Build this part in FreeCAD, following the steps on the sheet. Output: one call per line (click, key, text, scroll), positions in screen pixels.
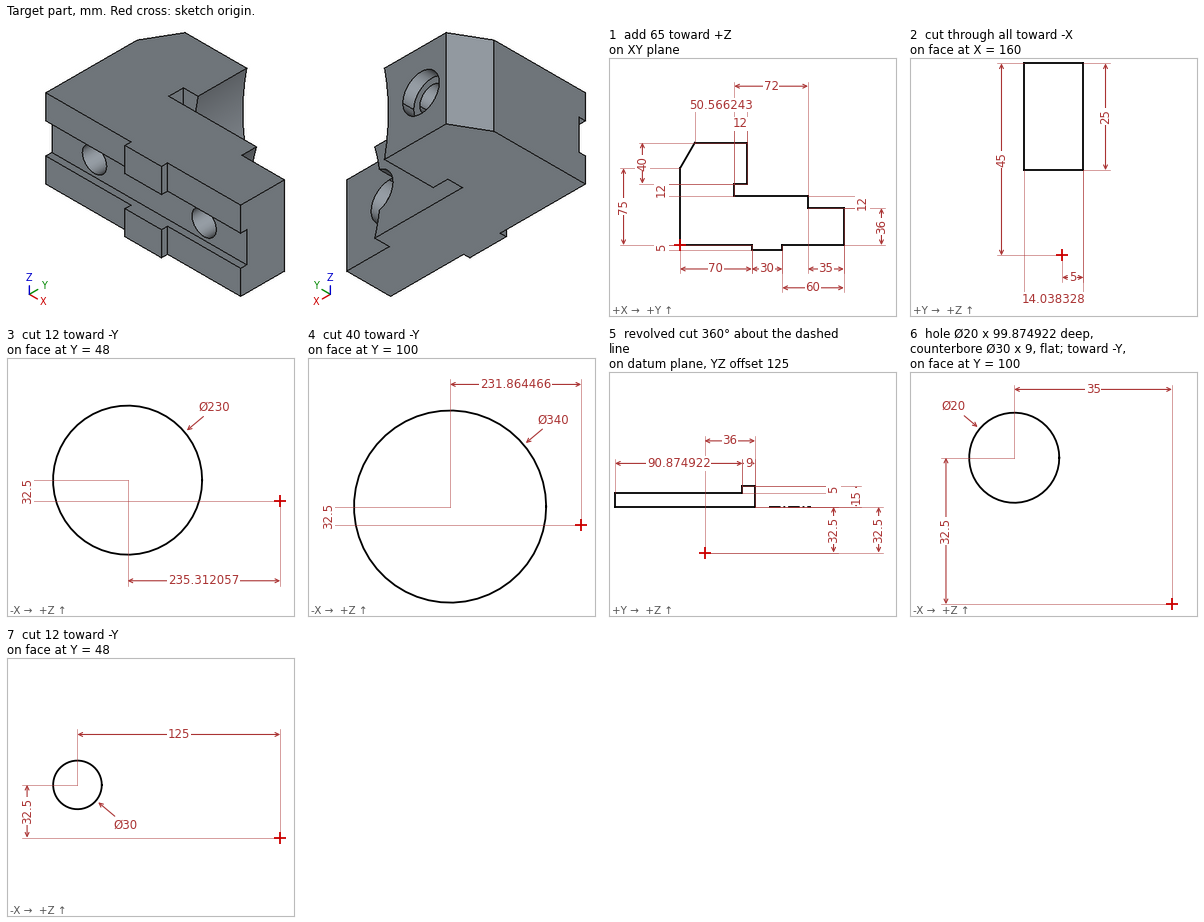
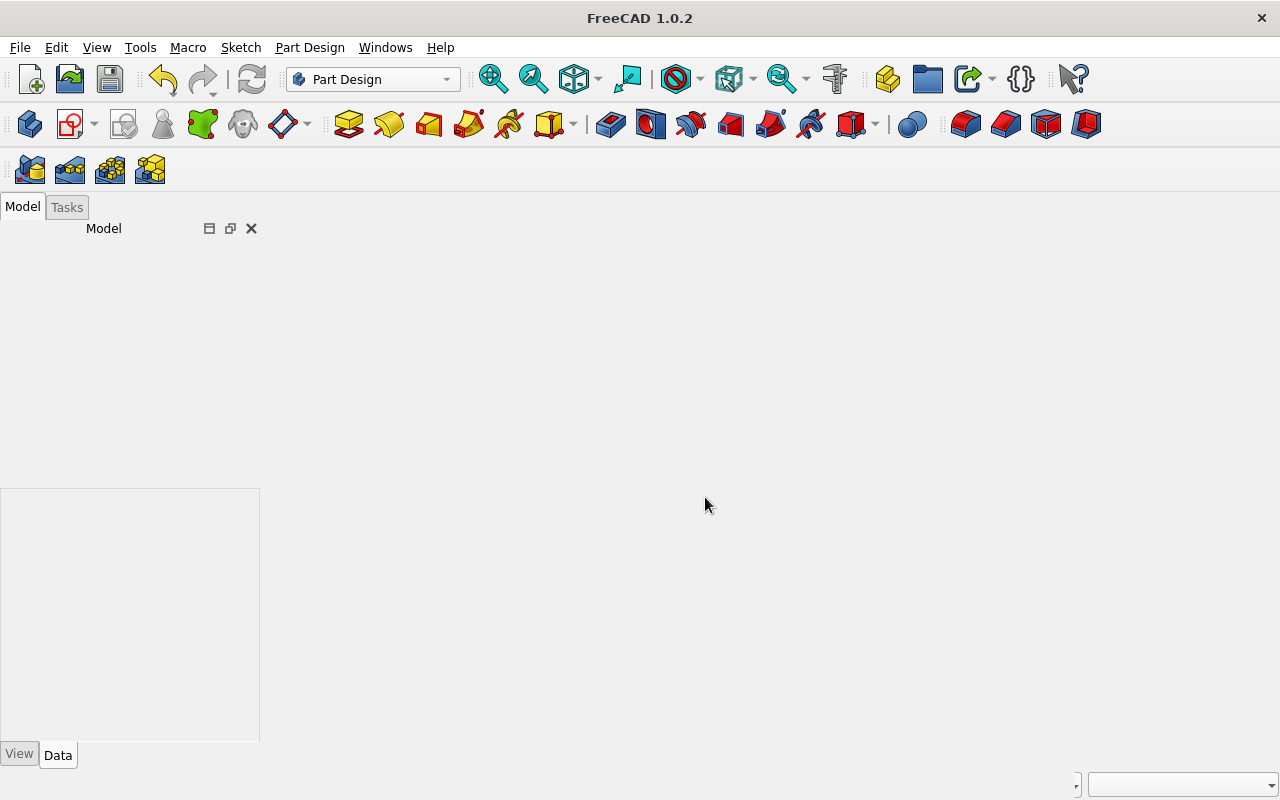
click(30, 80)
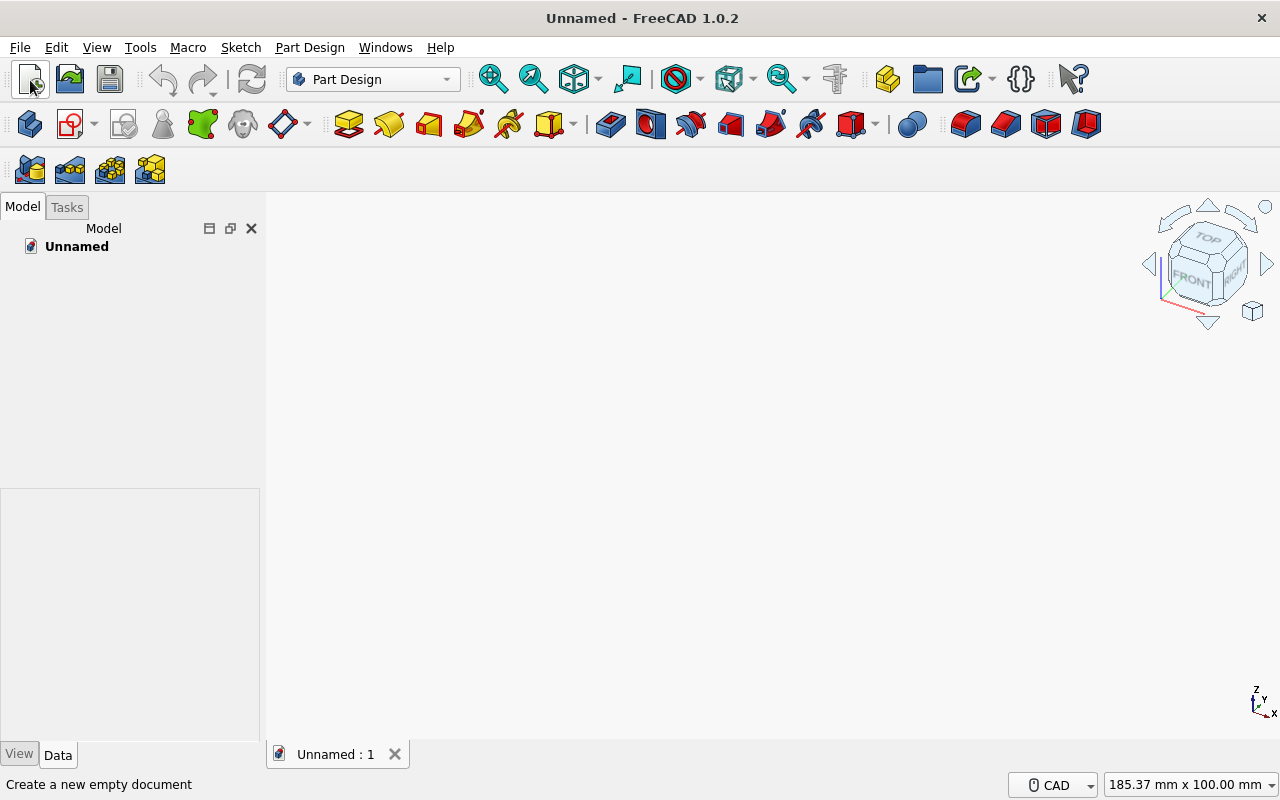
click(70, 124)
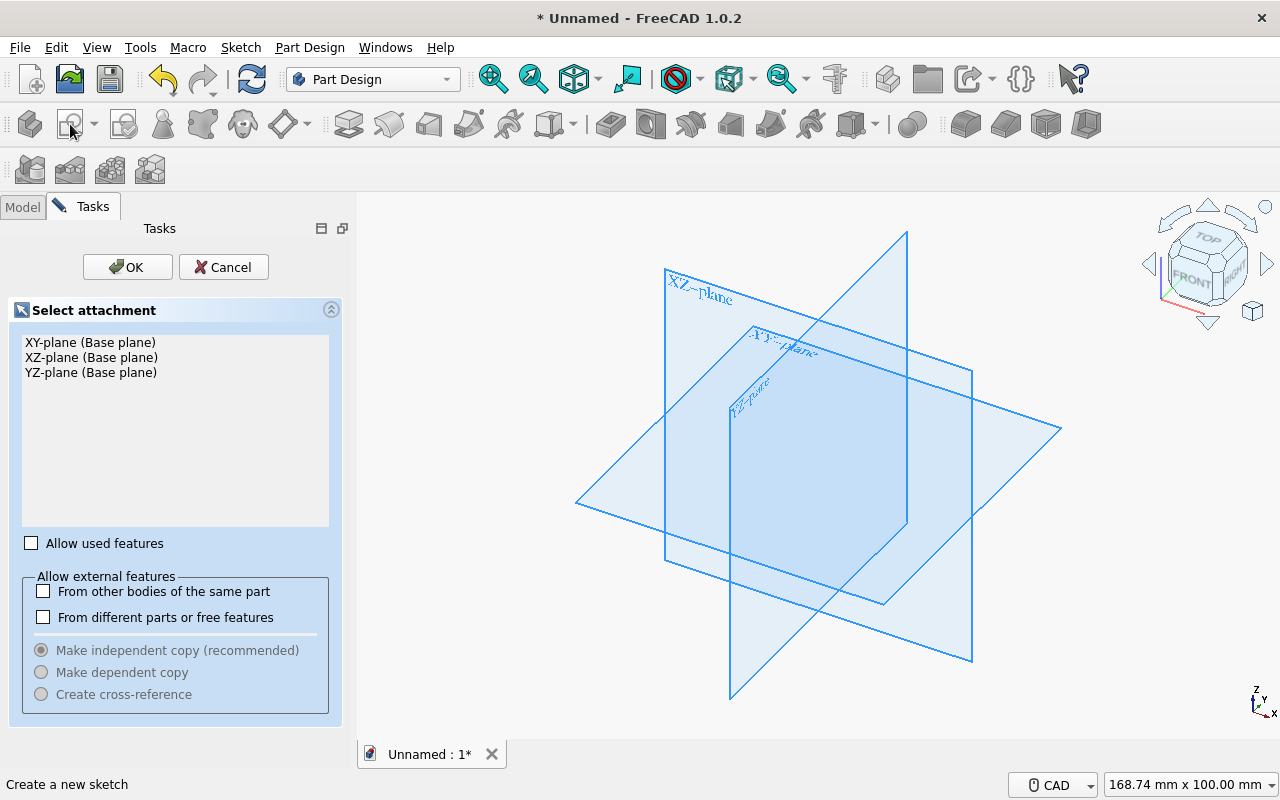
click(82, 342)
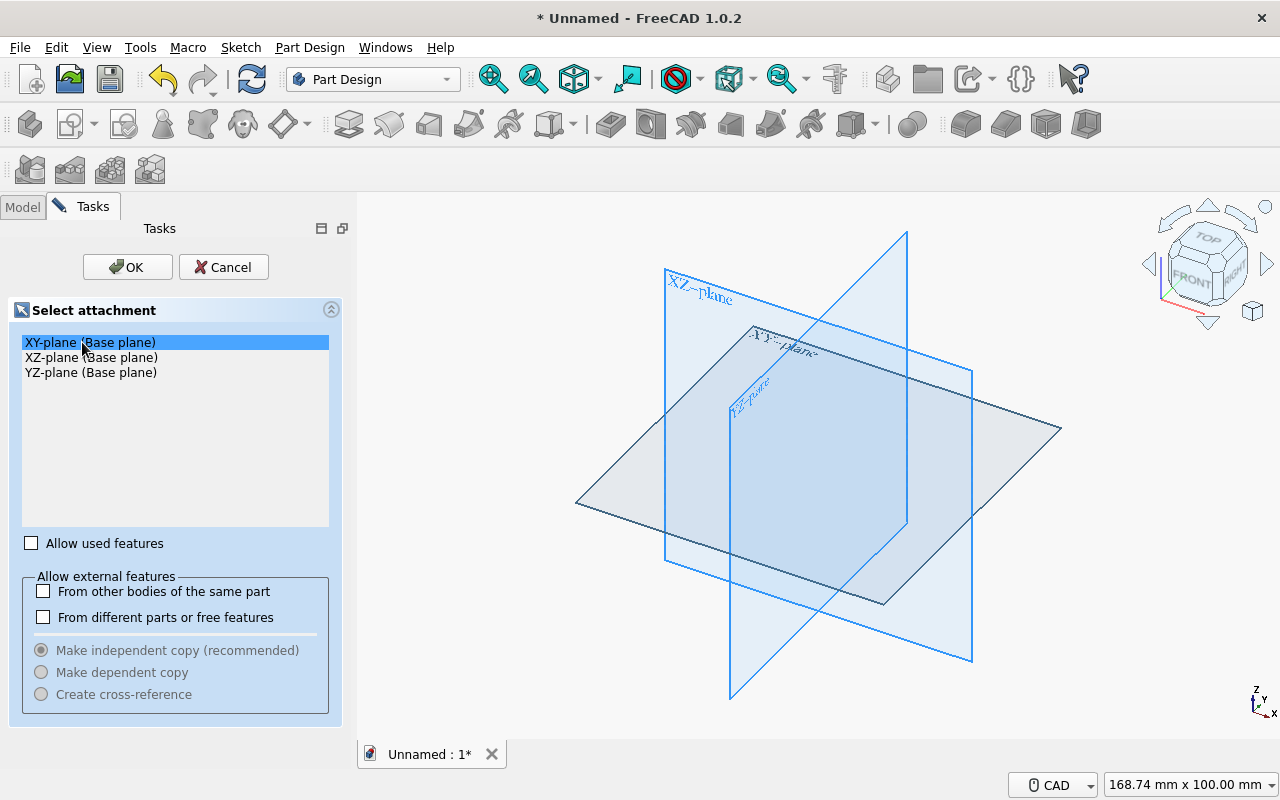
click(128, 267)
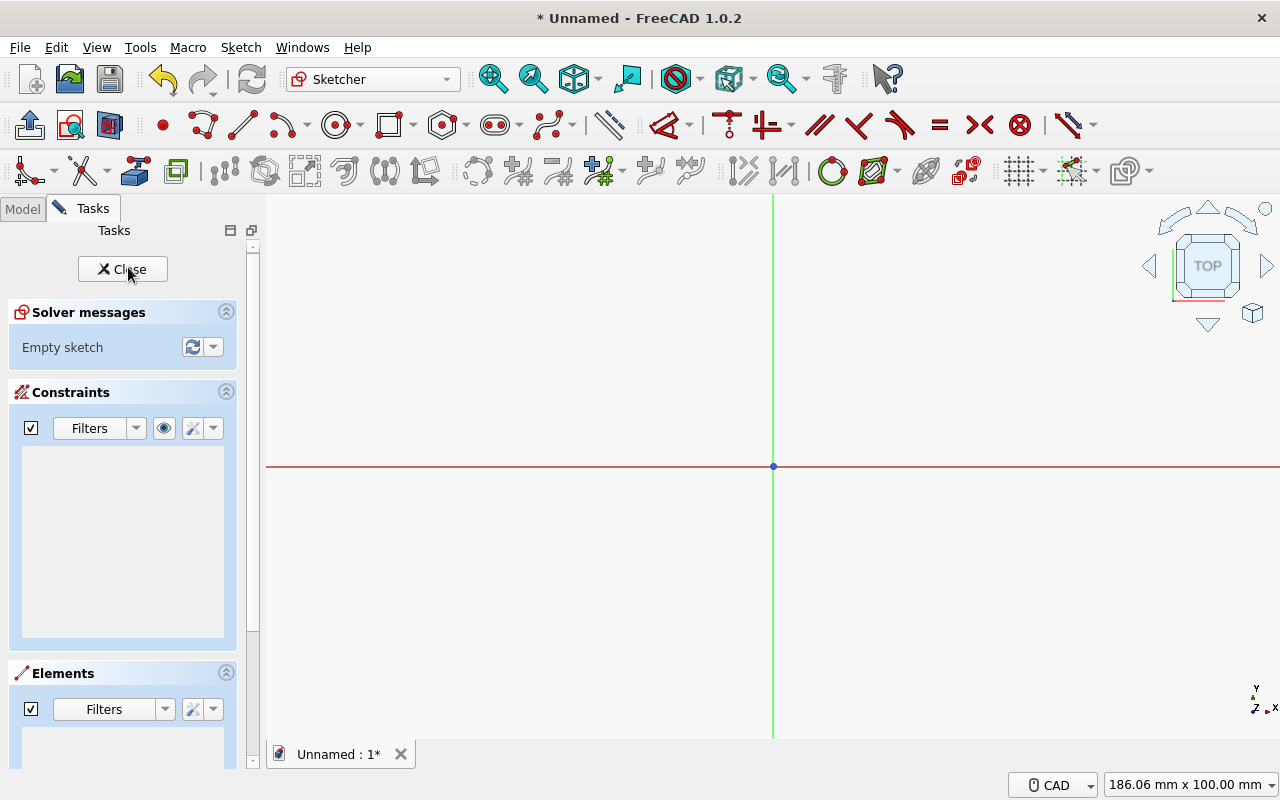
scroll(294, 711, down, 3)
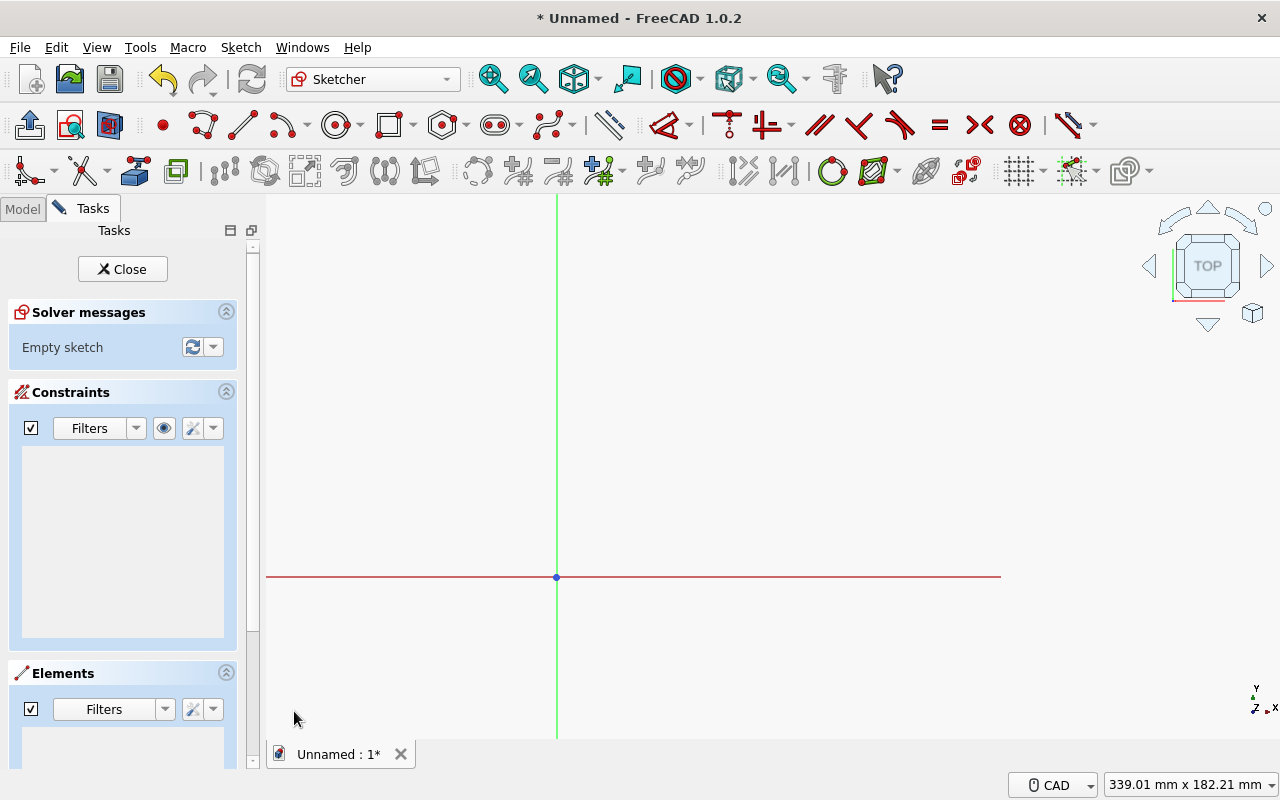
click(204, 126)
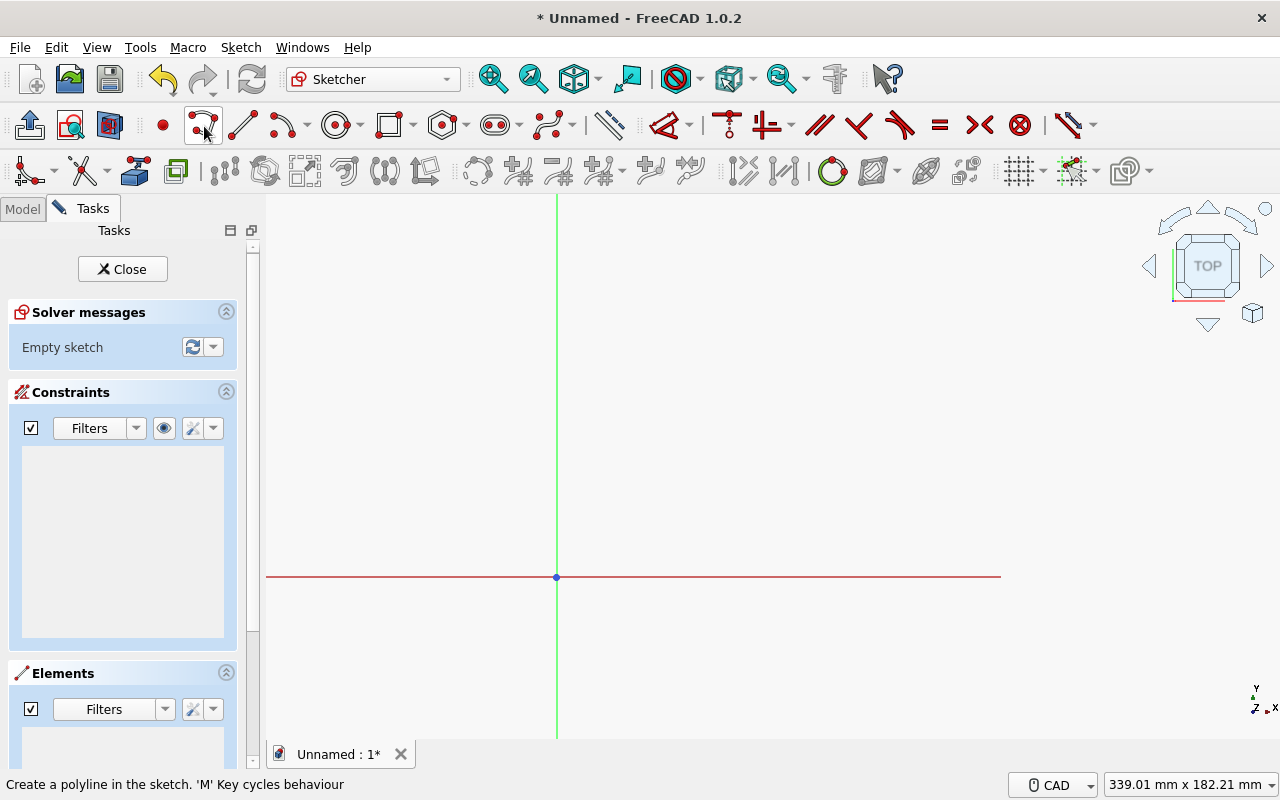
click(557, 577)
click(766, 568)
click(766, 592)
click(856, 592)
click(856, 577)
click(1035, 568)
click(1035, 470)
click(931, 470)
click(931, 434)
click(715, 434)
click(715, 398)
click(751, 398)
click(751, 278)
click(600, 278)
click(566, 353)
click(557, 577)
key(Escape)
key(Escape)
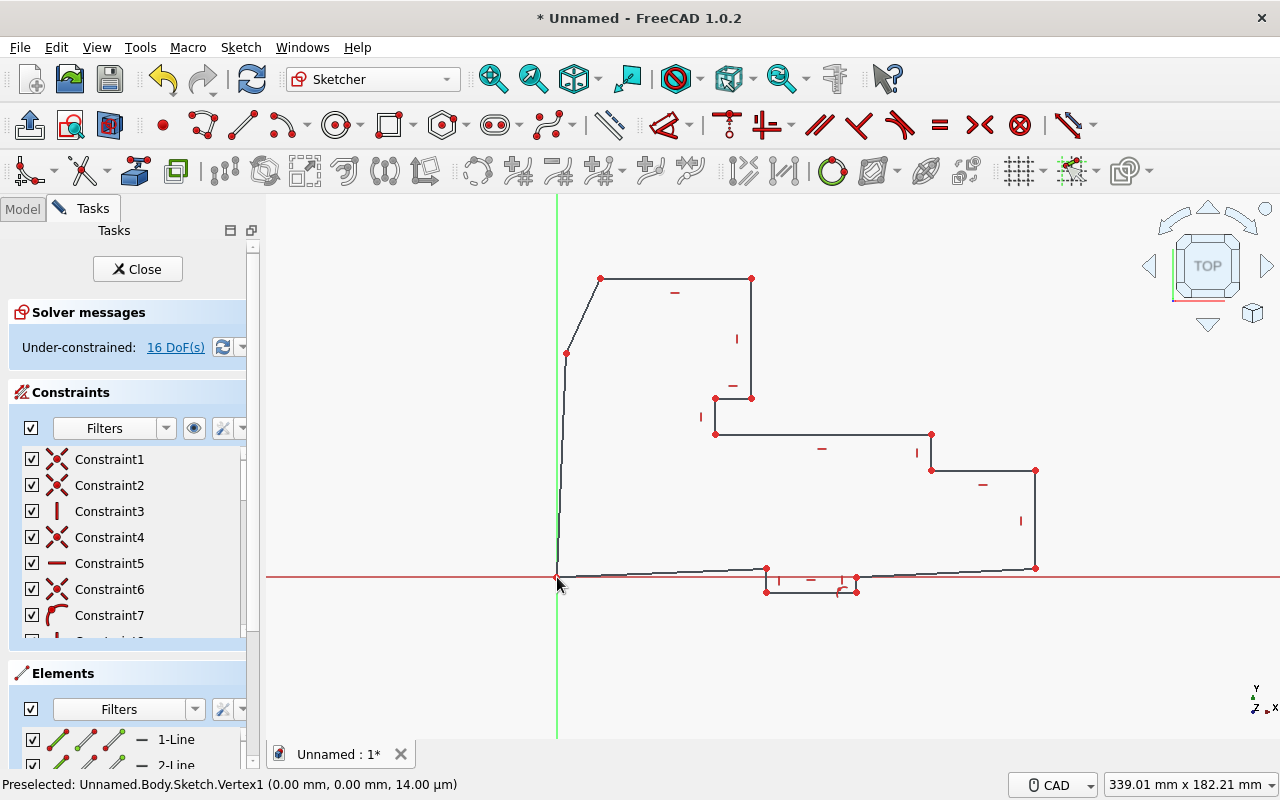
click(620, 575)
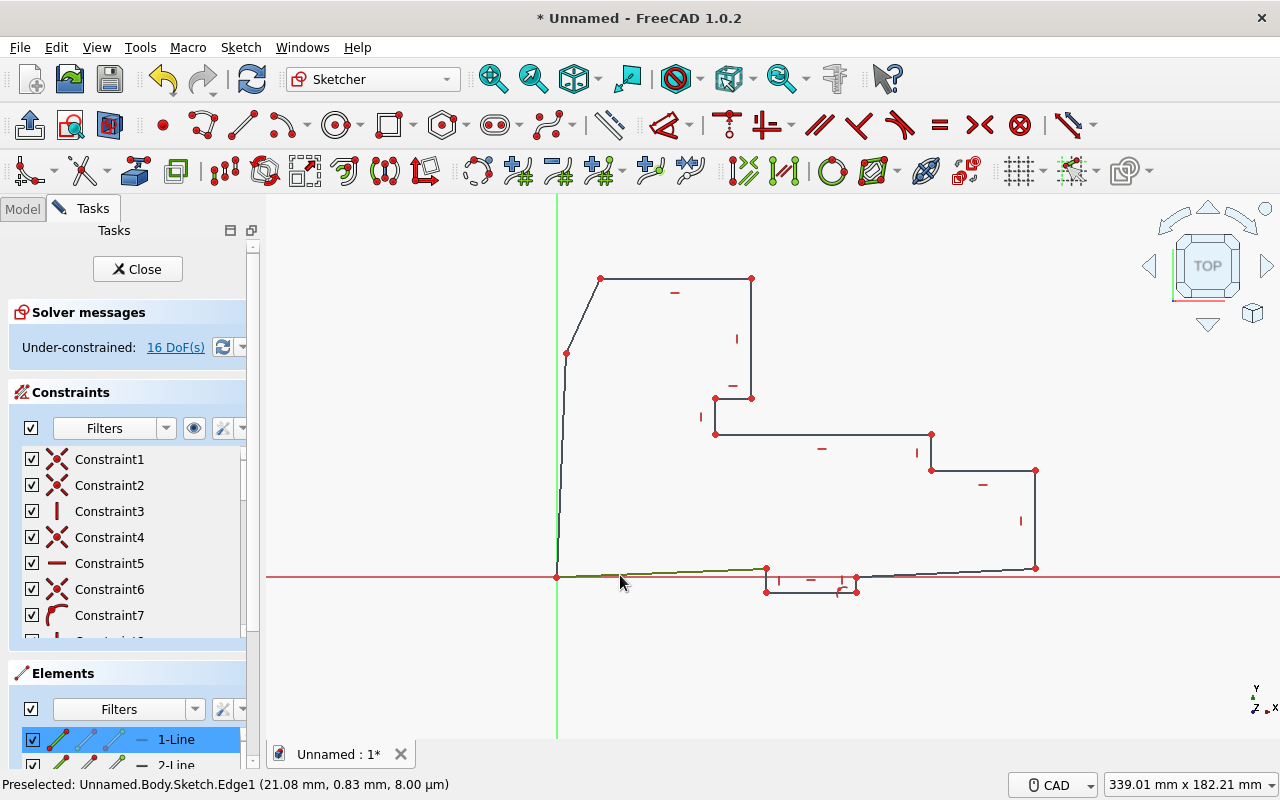
click(794, 126)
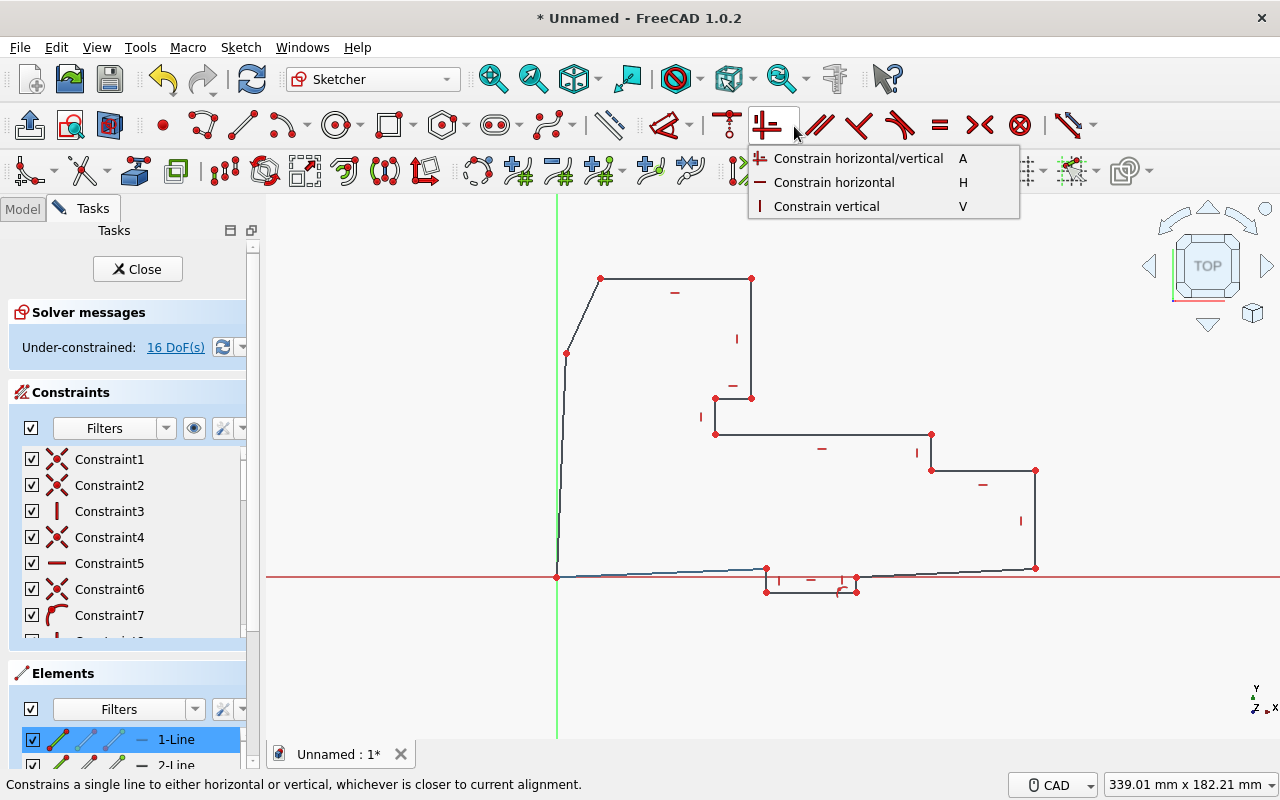
click(884, 182)